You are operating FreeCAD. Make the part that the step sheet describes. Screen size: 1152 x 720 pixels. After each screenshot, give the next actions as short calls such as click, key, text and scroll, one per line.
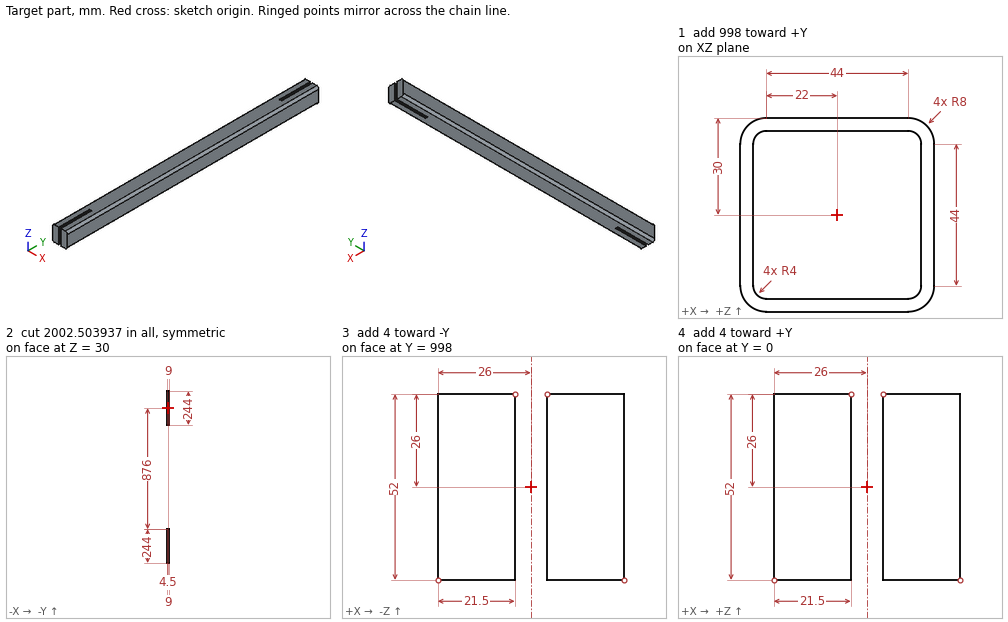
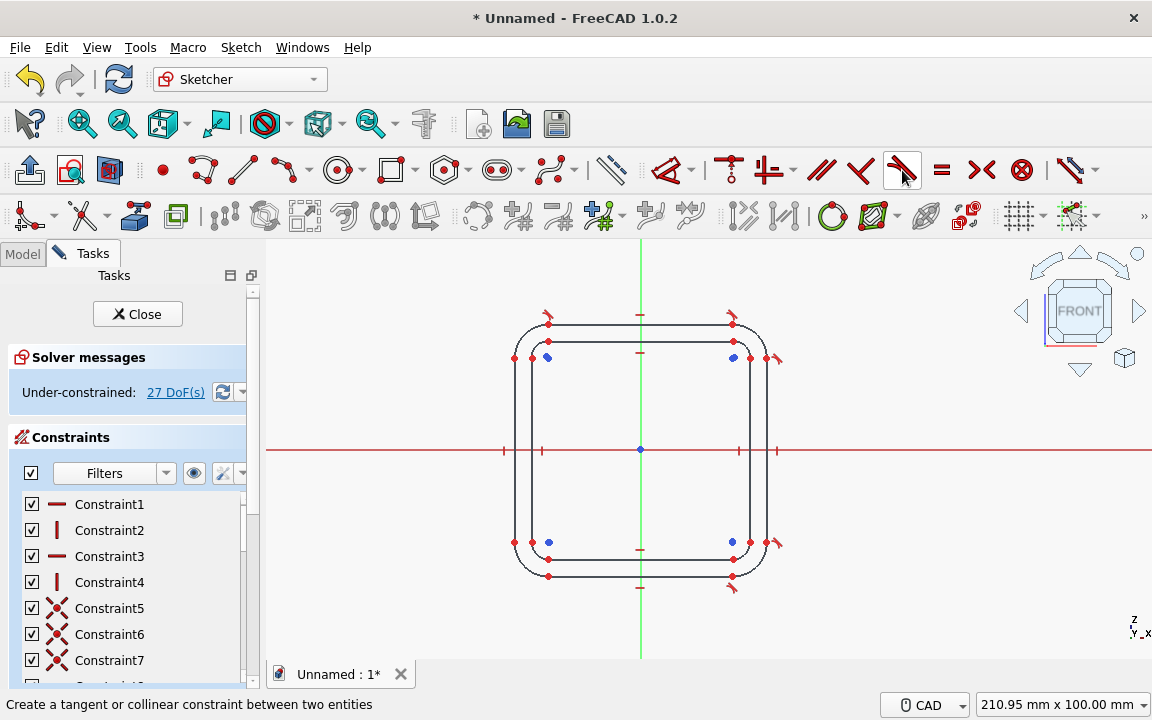
click(677, 577)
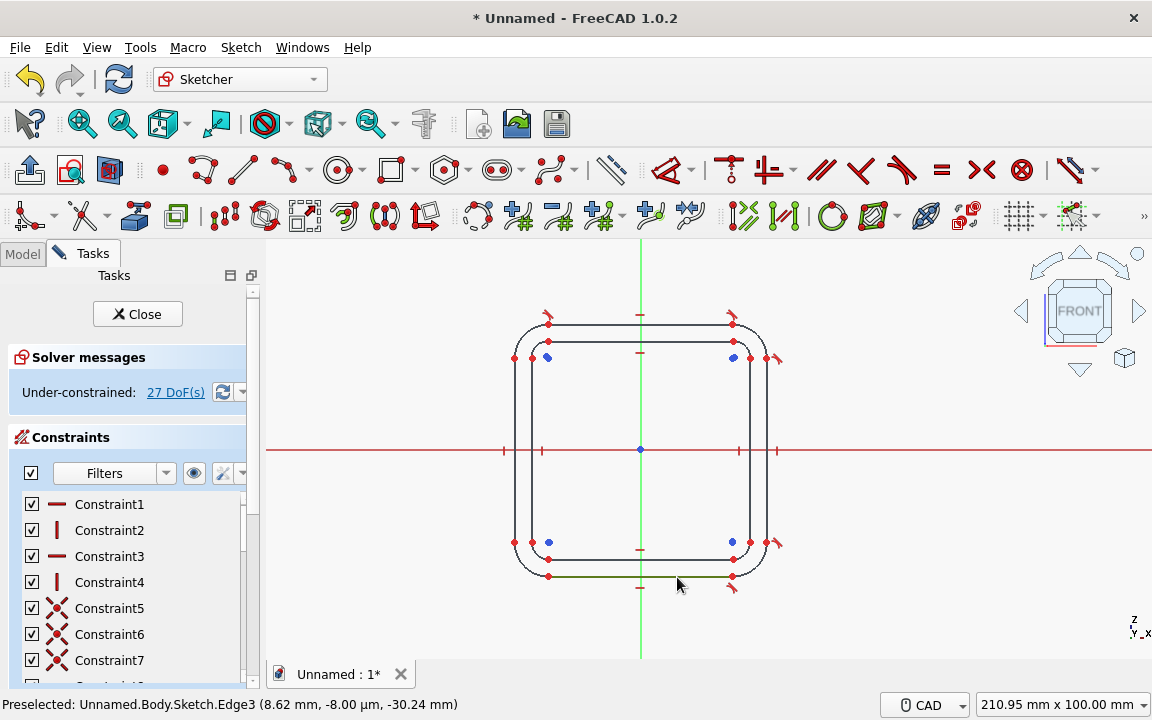
click(518, 558)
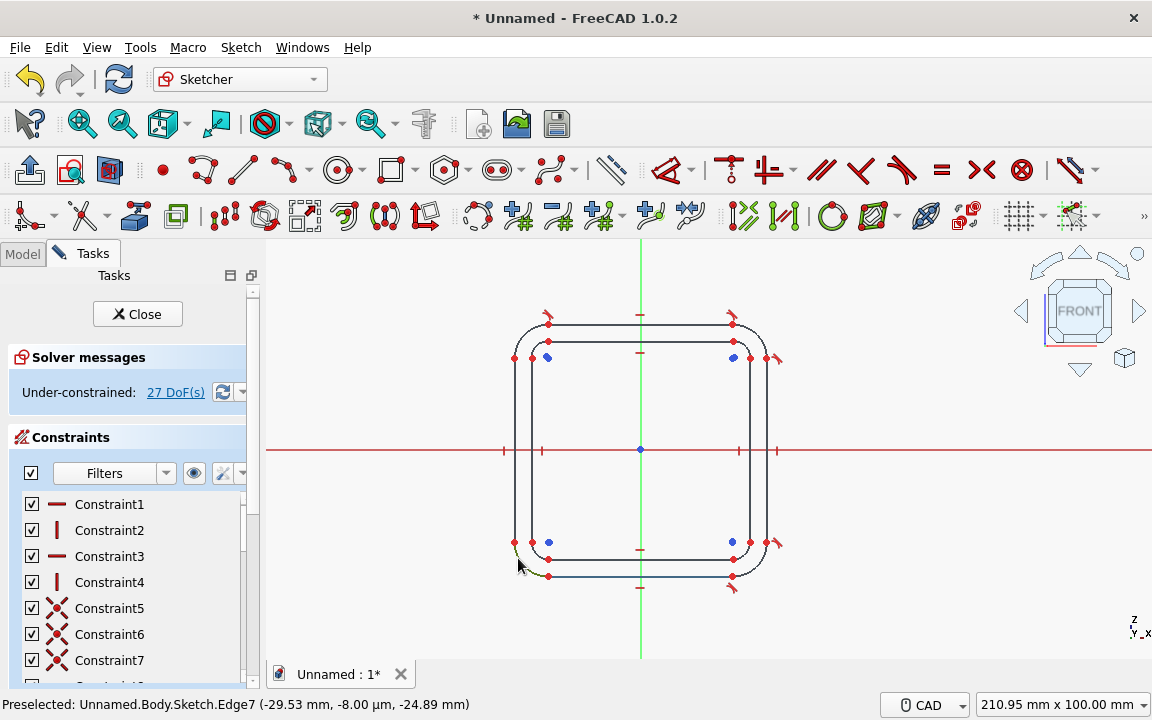
click(902, 170)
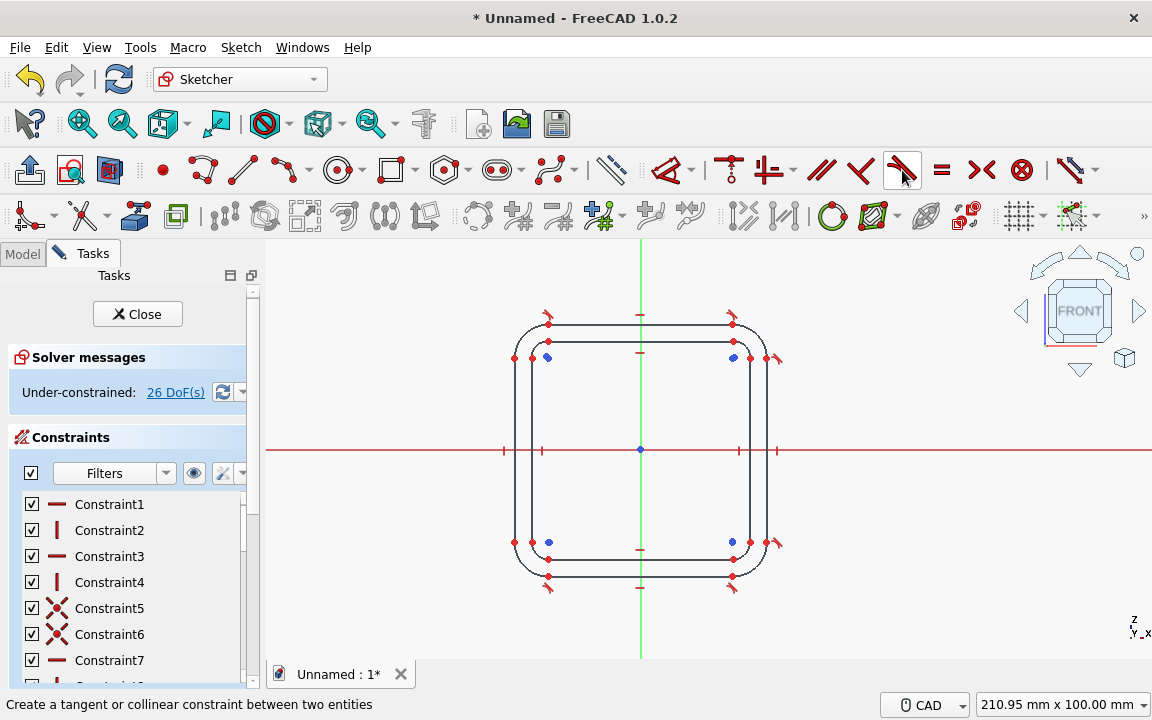
click(515, 488)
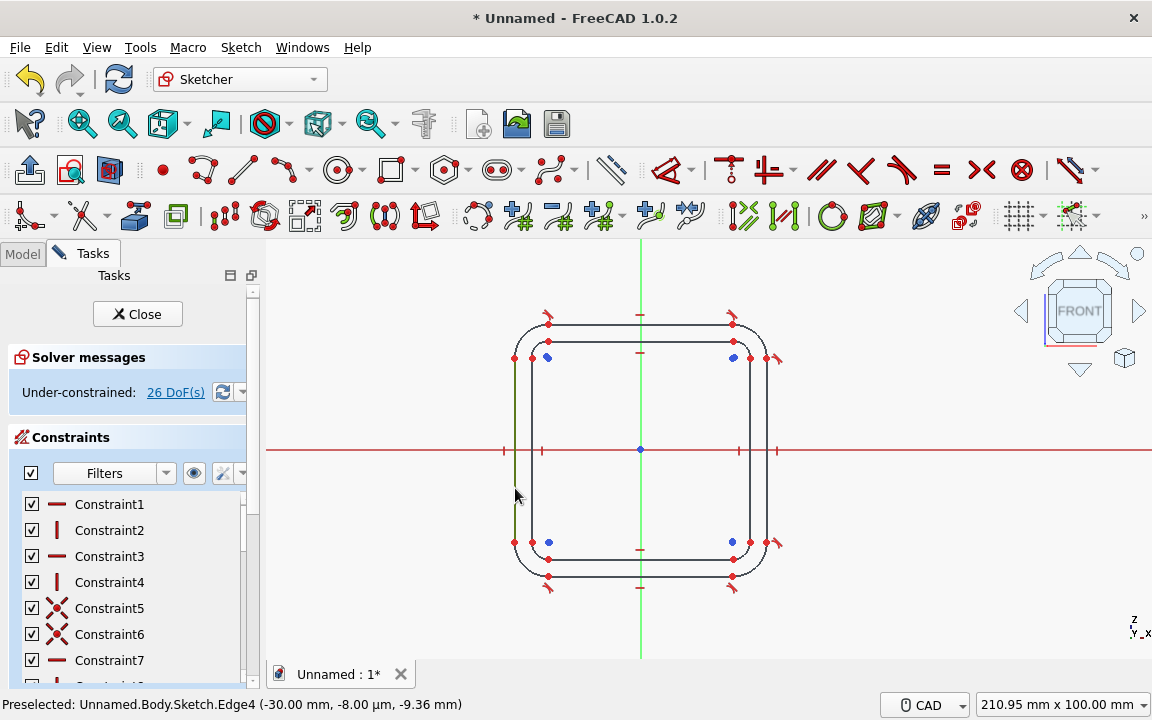
click(519, 558)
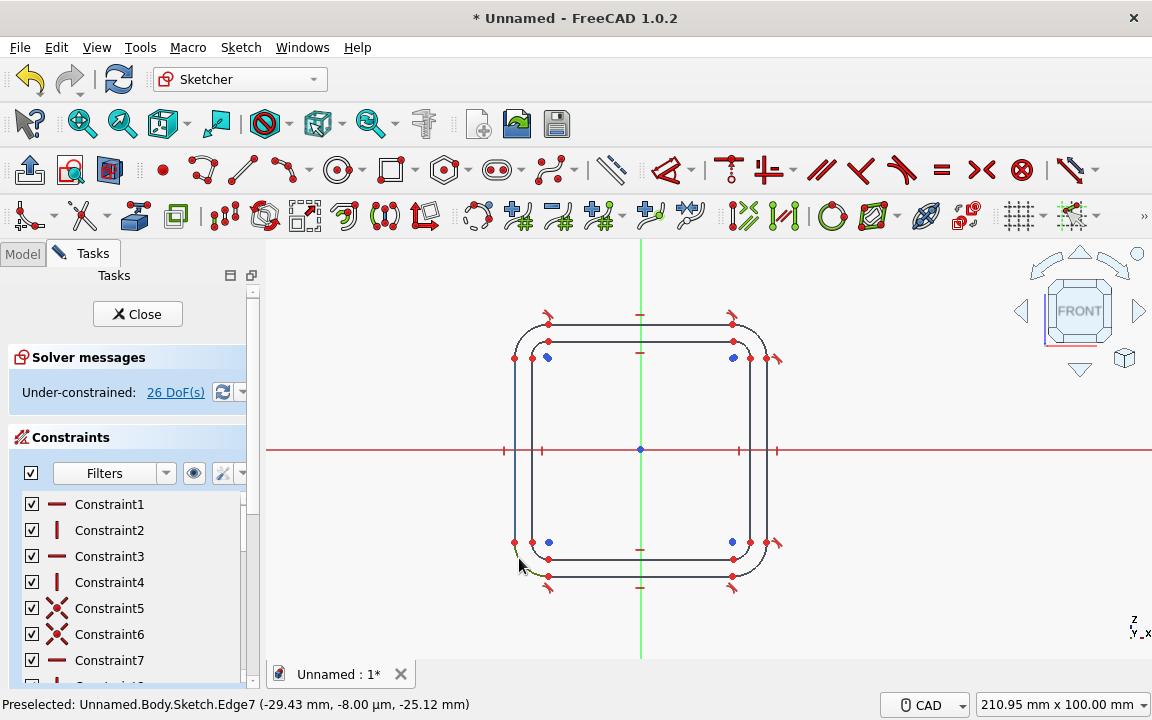
click(902, 170)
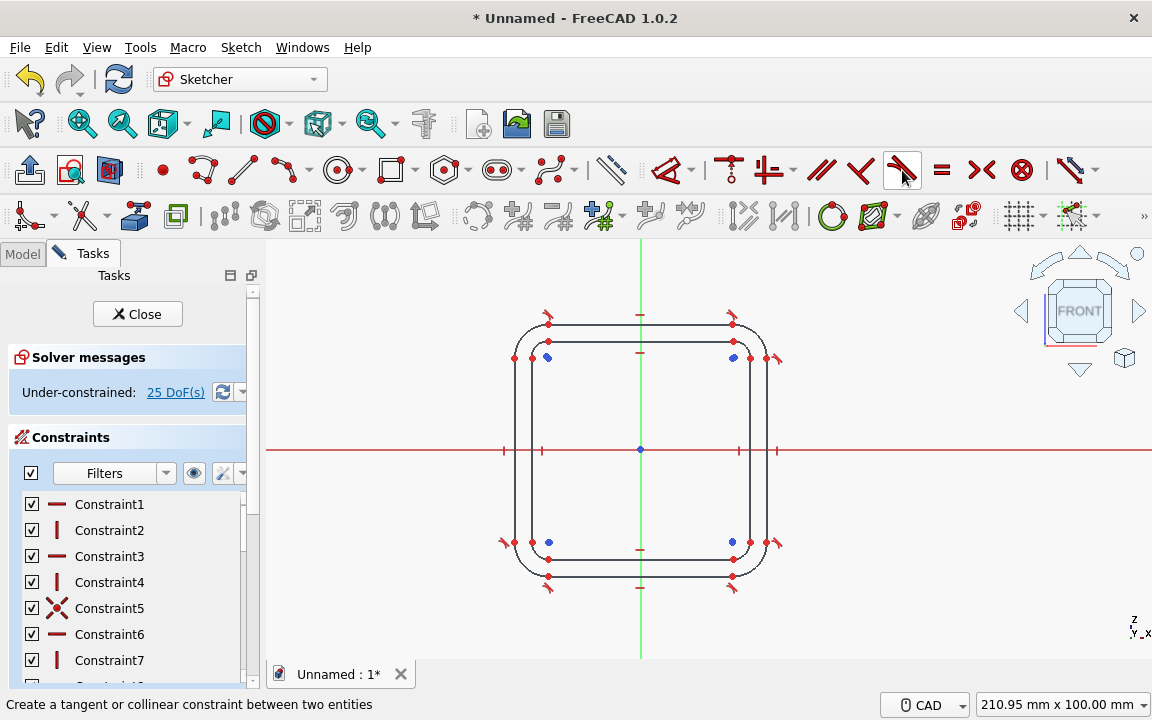
click(515, 488)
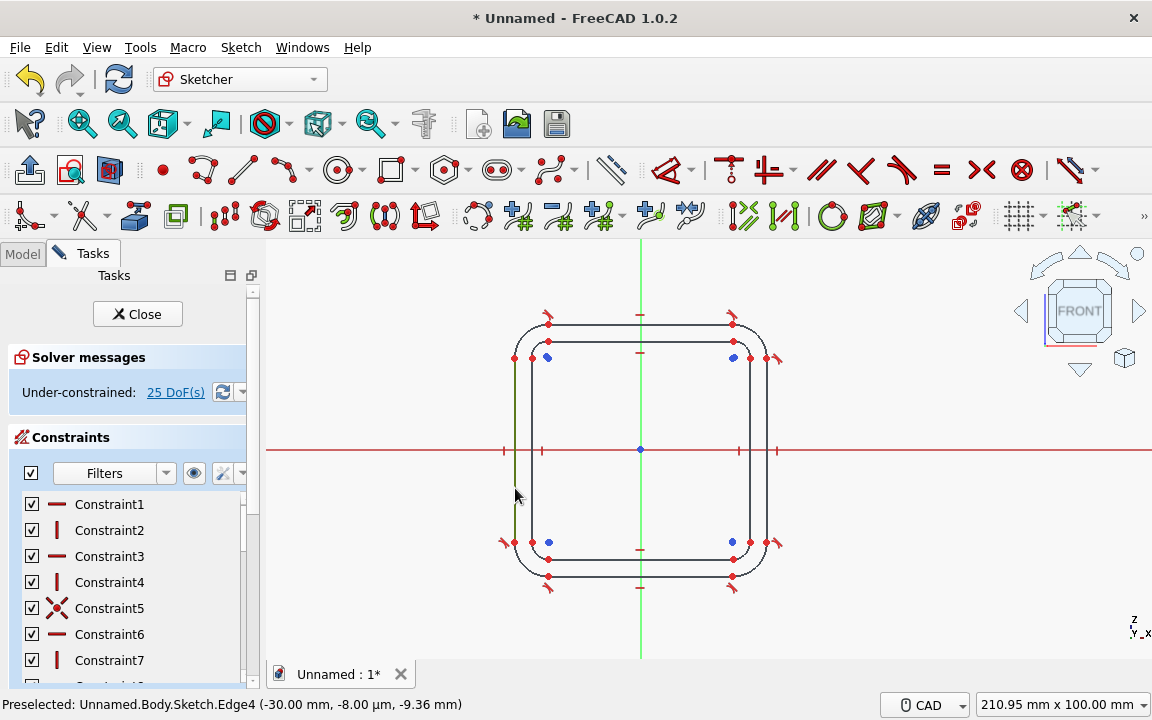
click(533, 328)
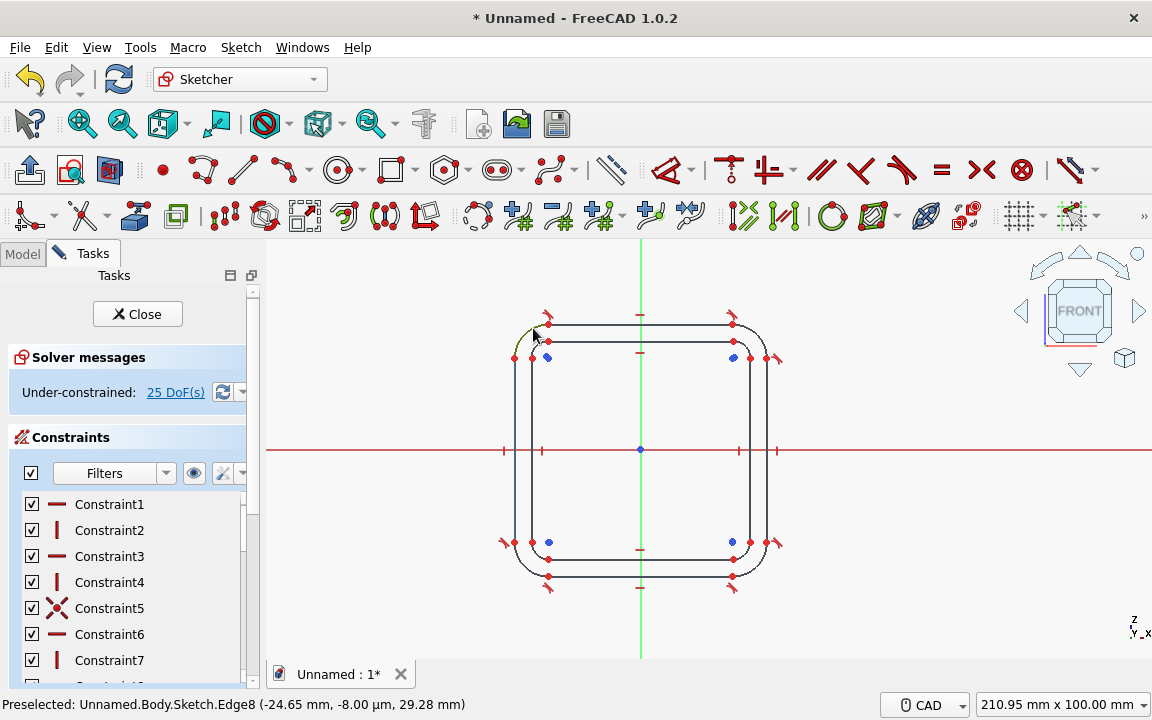
key(t)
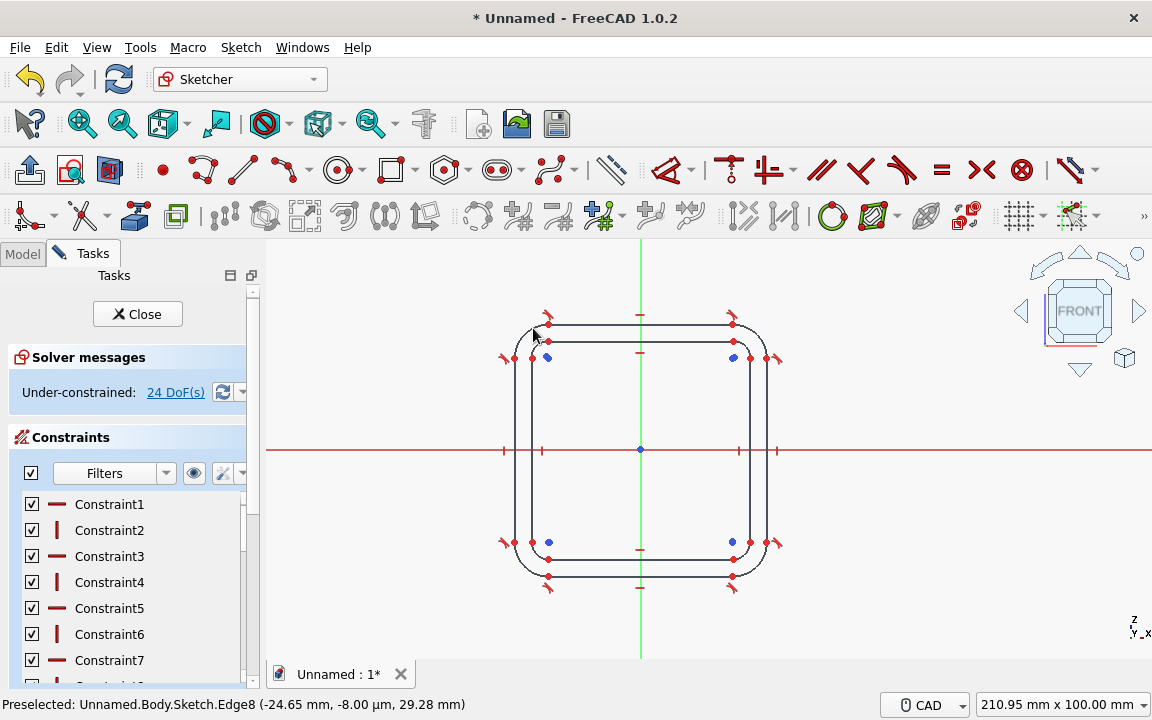
click(604, 560)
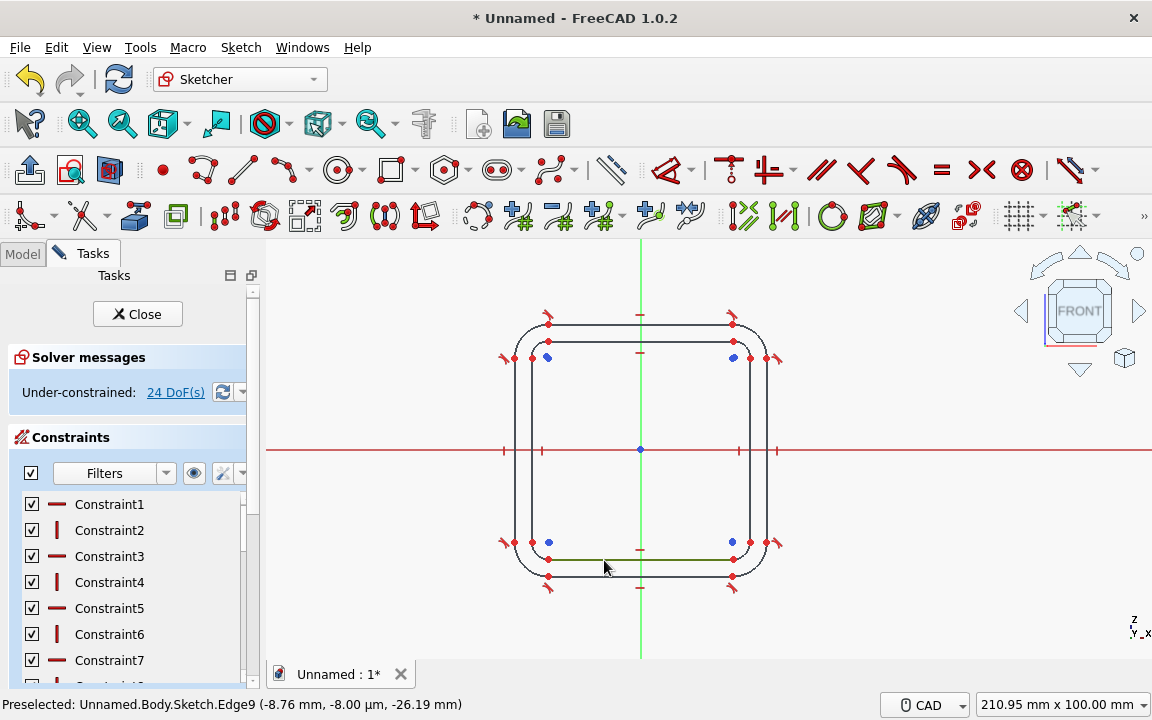
click(745, 555)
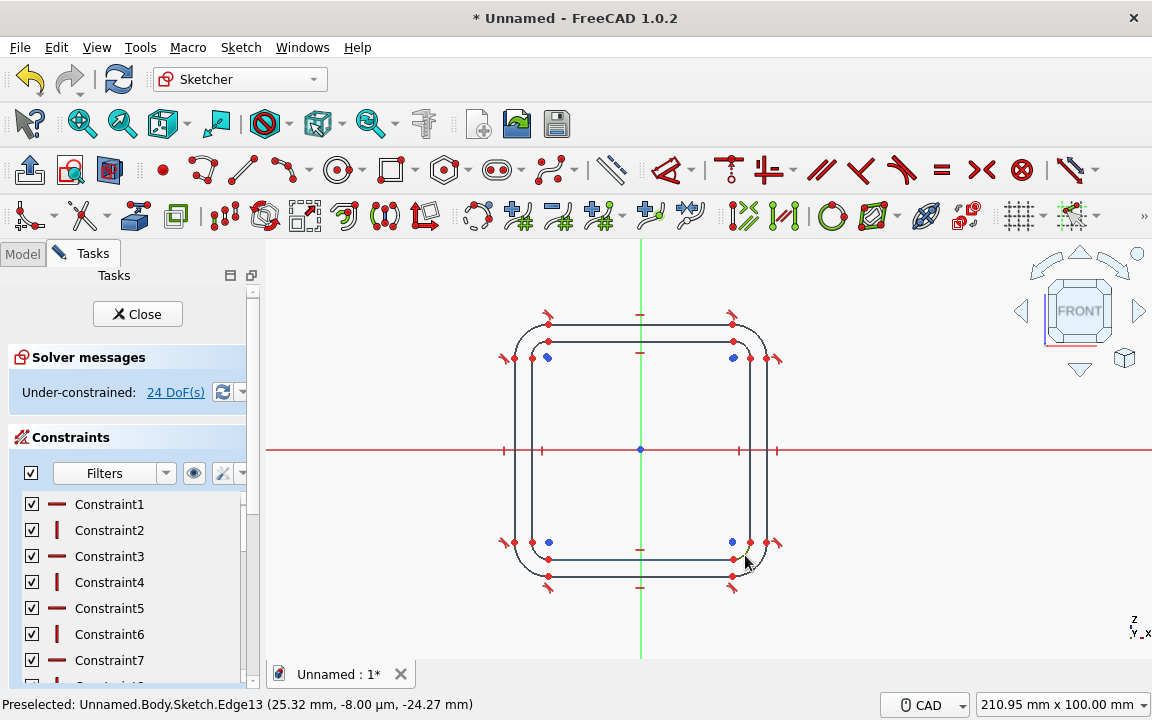
click(902, 170)